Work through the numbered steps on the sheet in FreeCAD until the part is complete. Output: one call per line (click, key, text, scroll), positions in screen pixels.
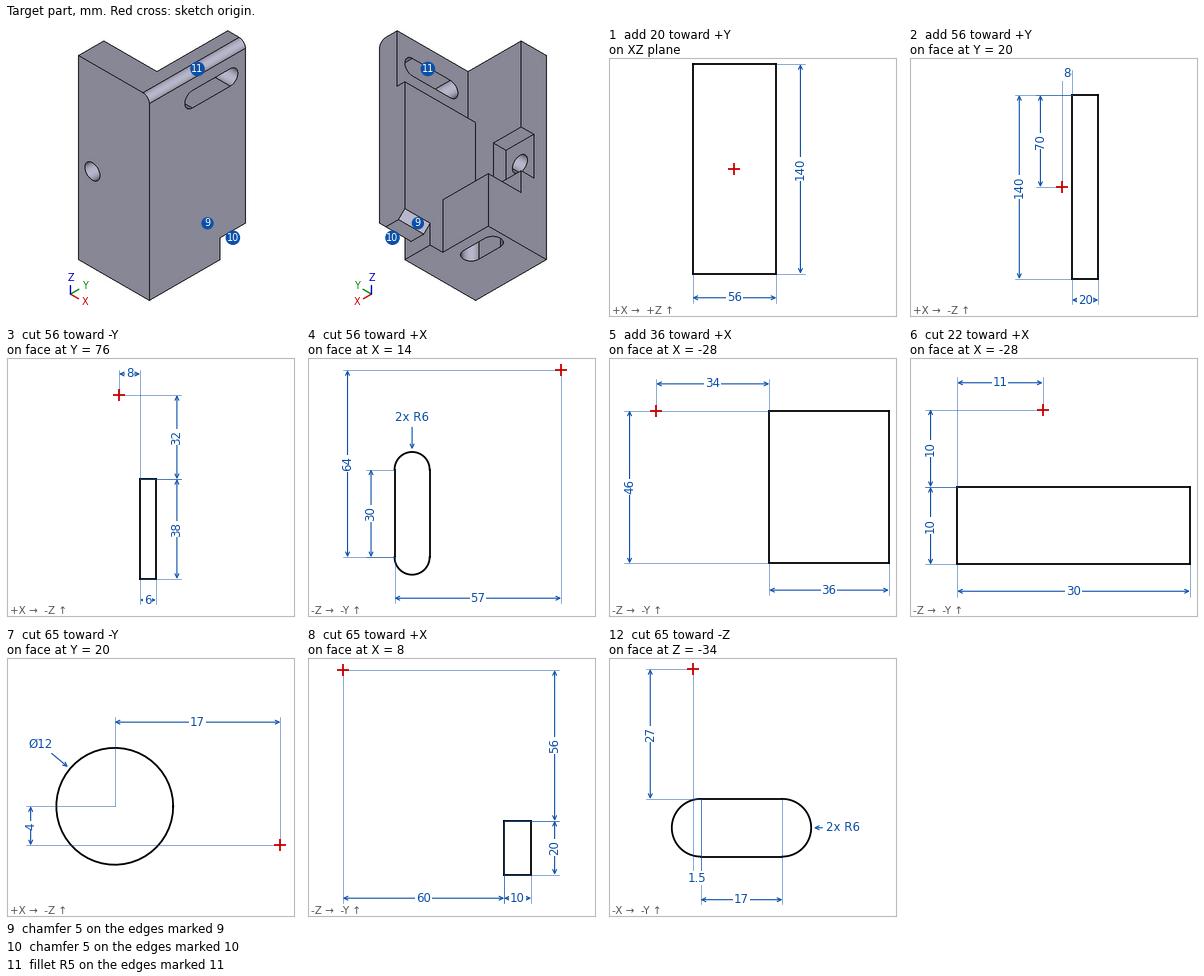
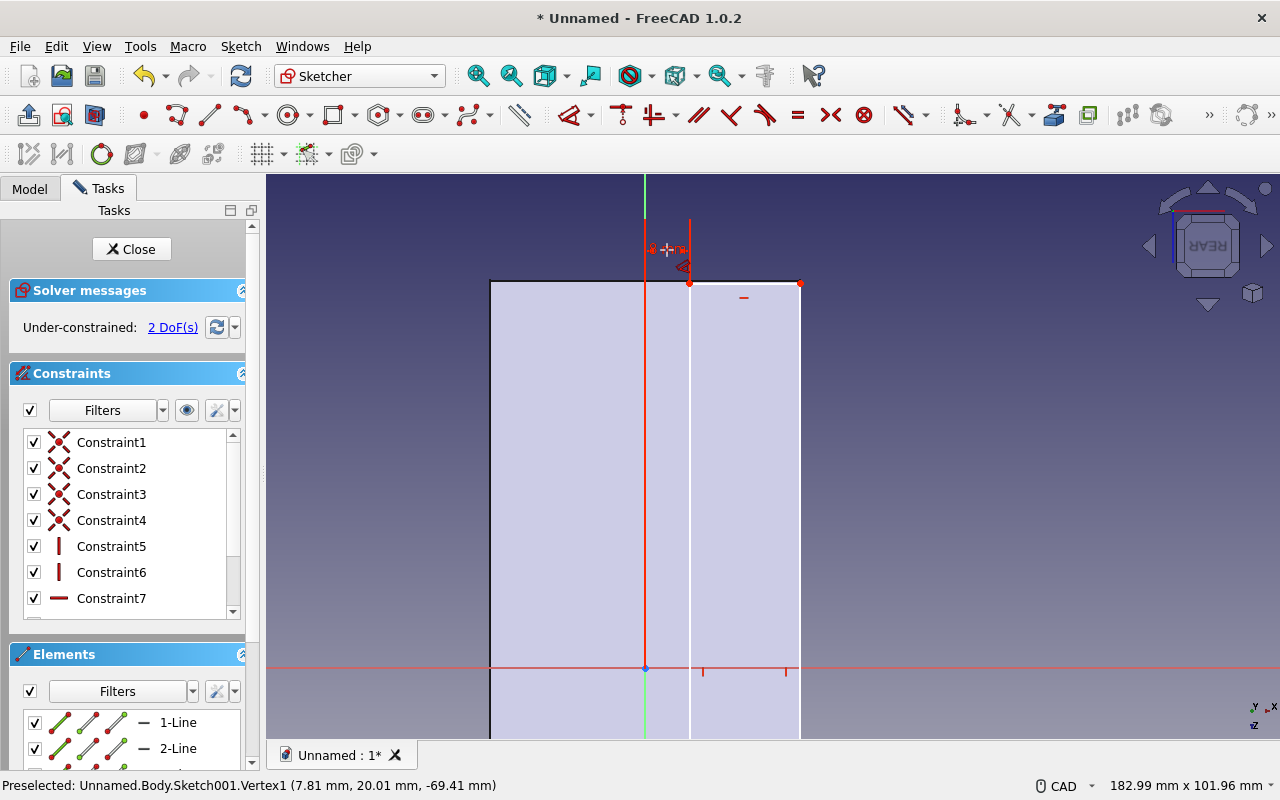
click(690, 516)
click(724, 497)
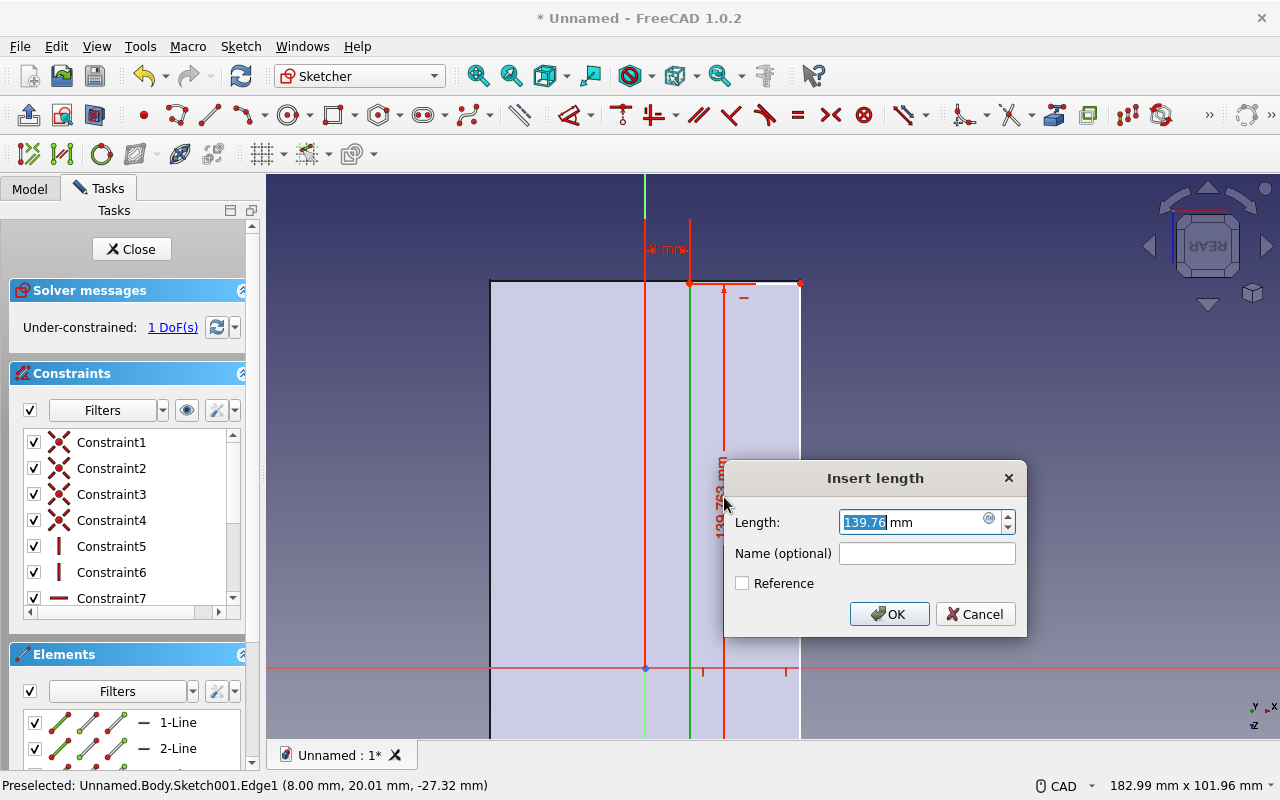
text(140)
key(Return)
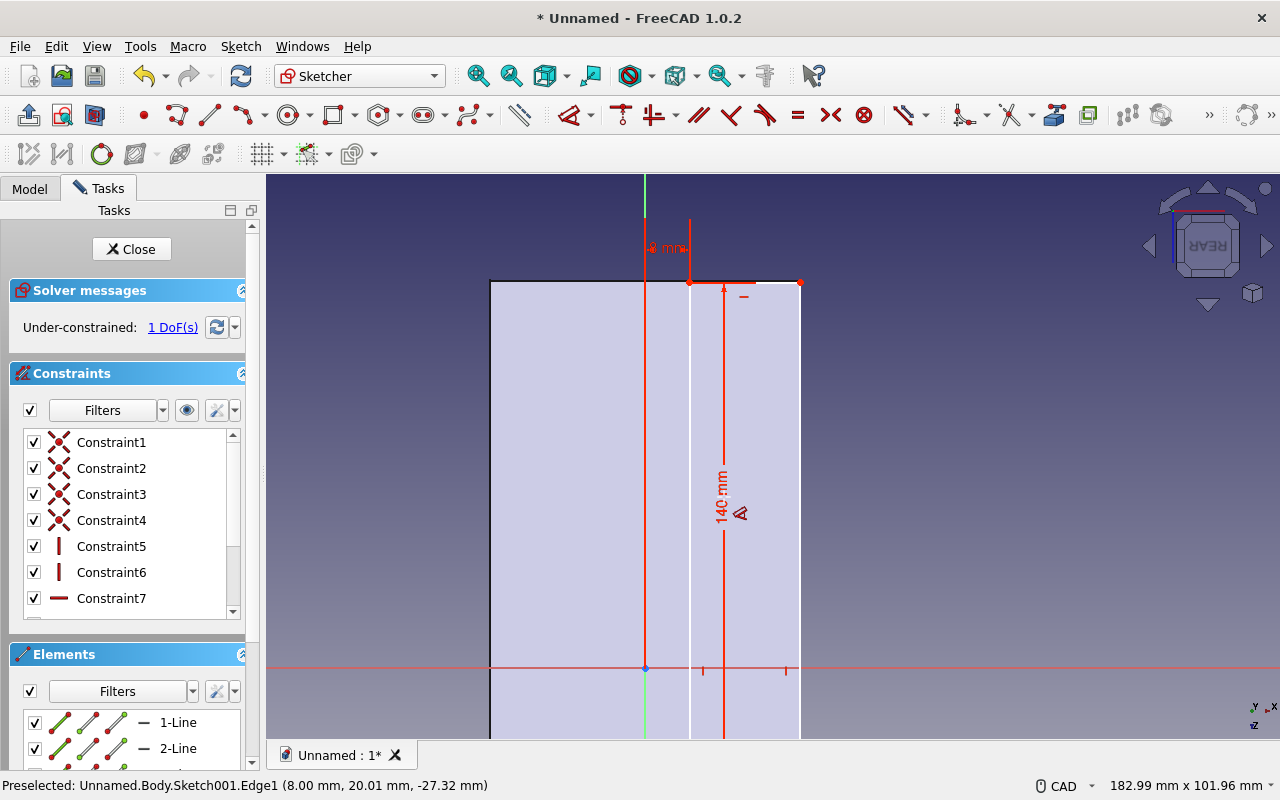
click(690, 283)
click(611, 476)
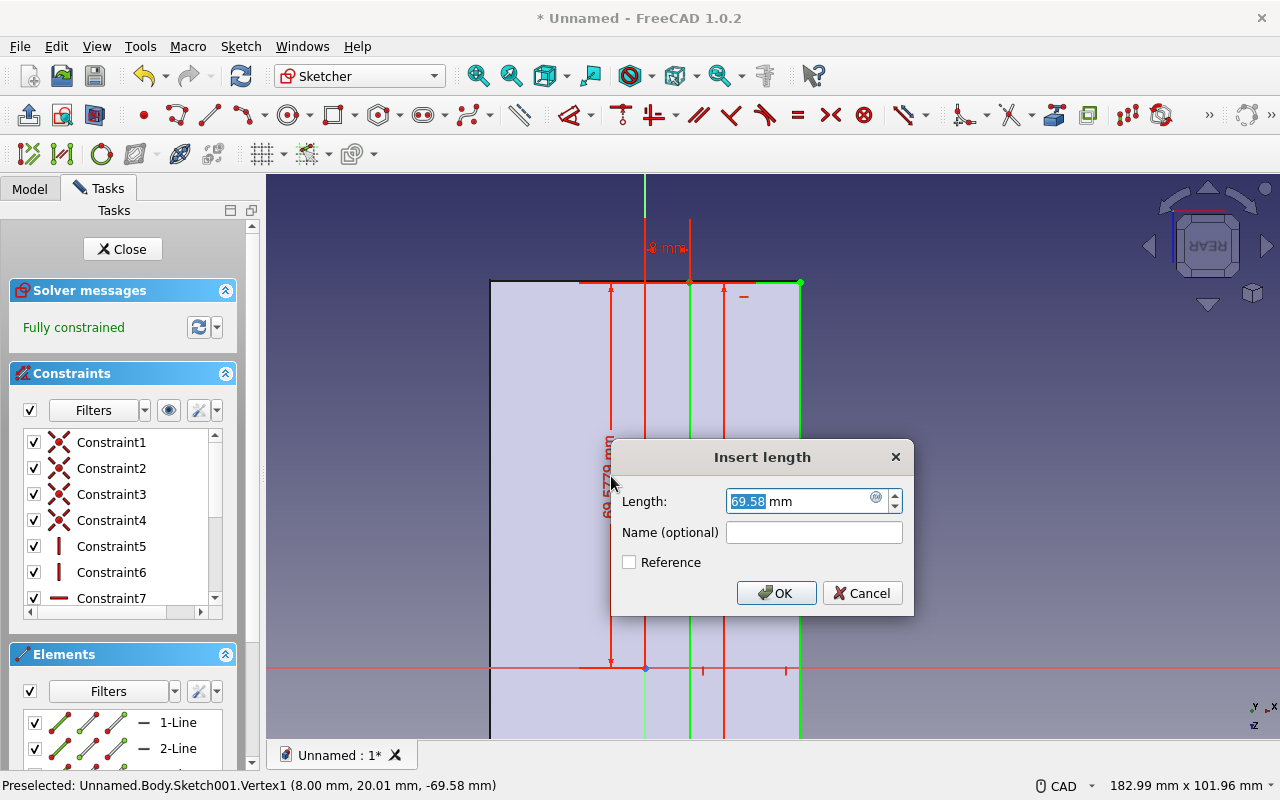
text(70)
key(Return)
key(Escape)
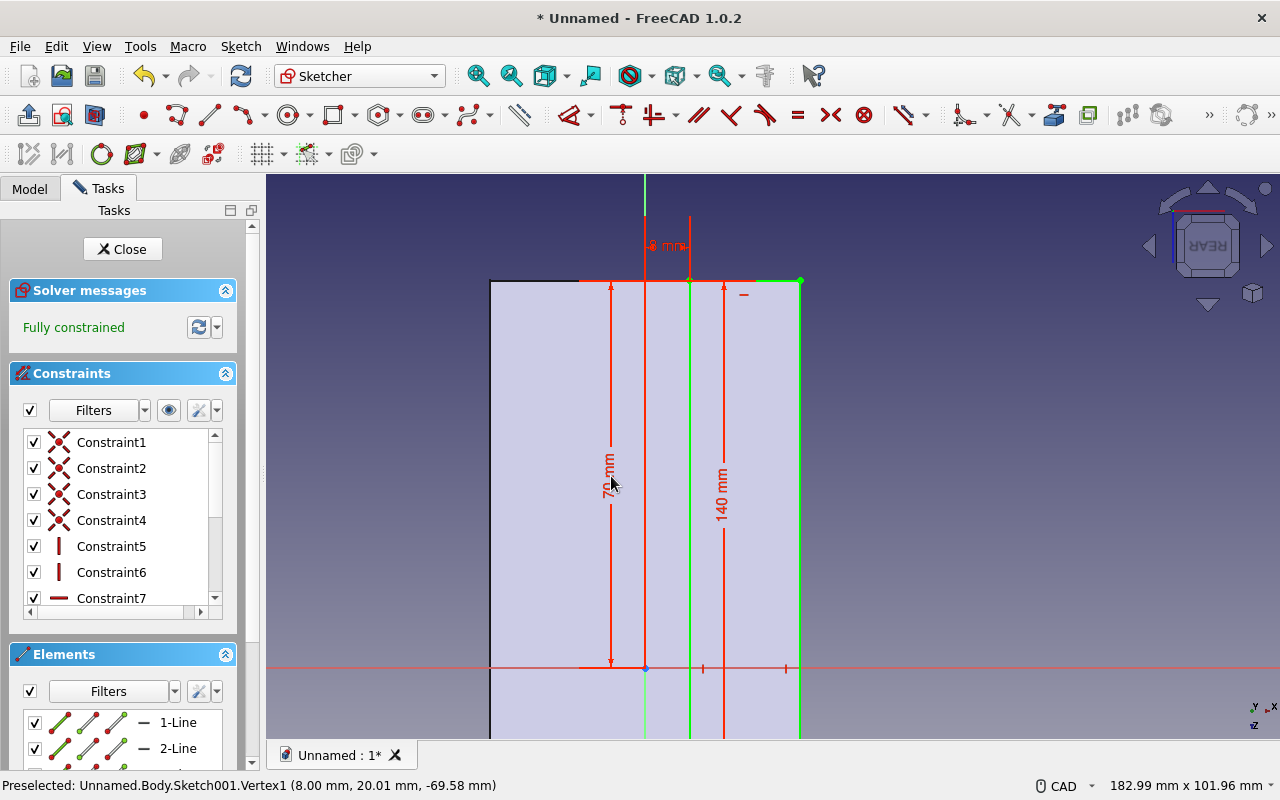
click(123, 249)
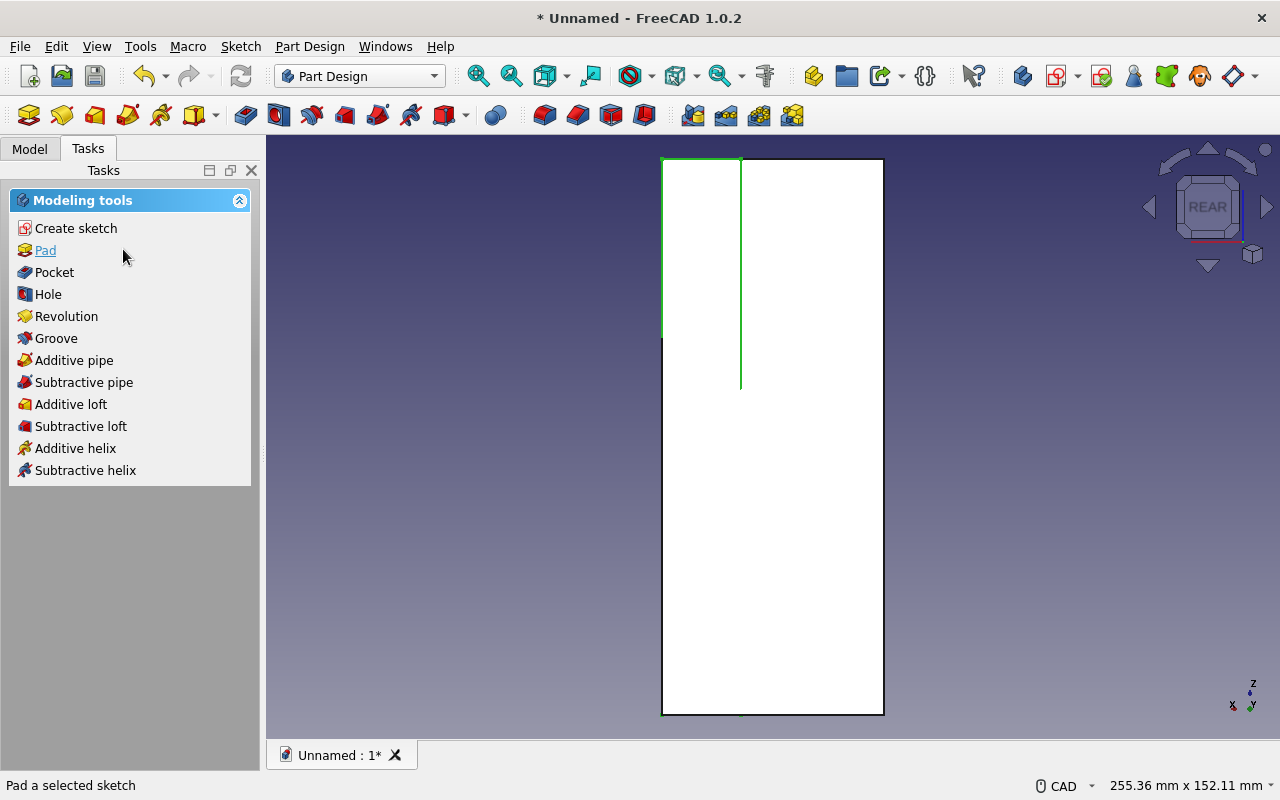
click(29, 116)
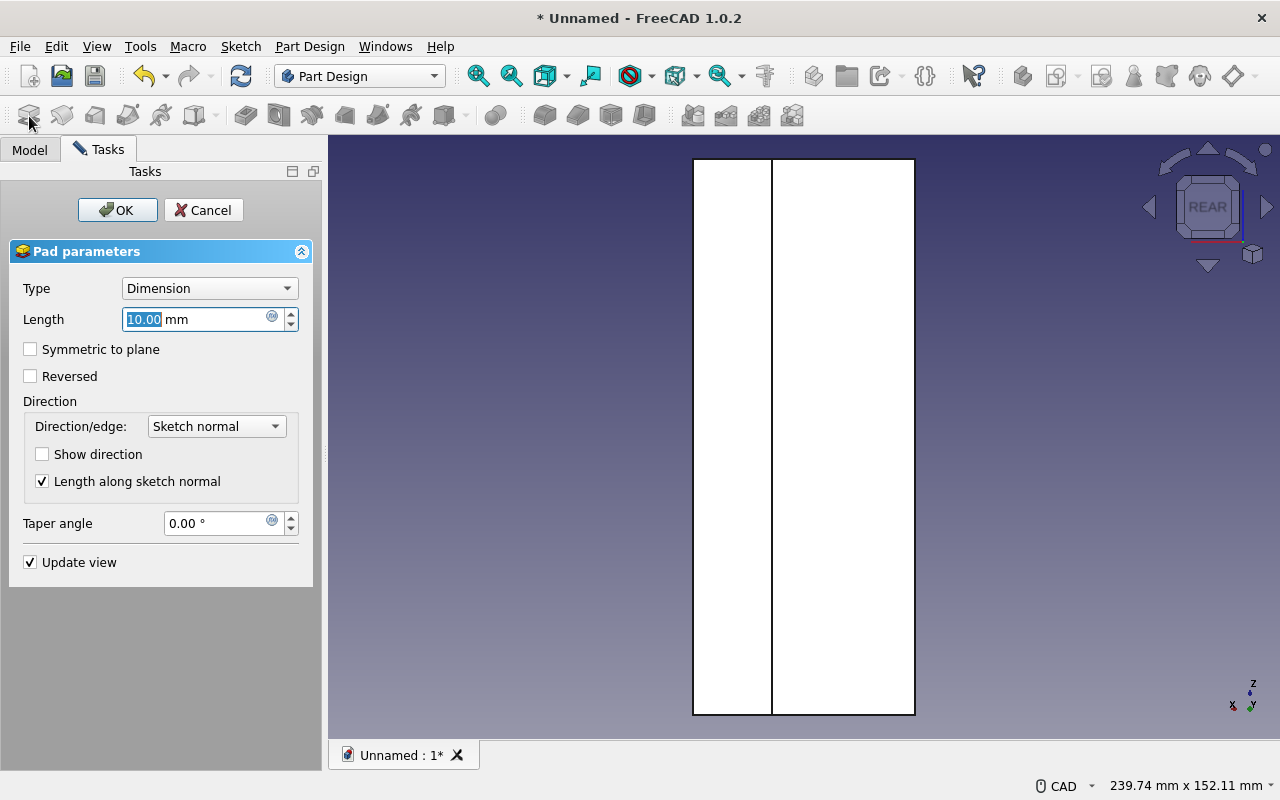
text(56)
key(Tab)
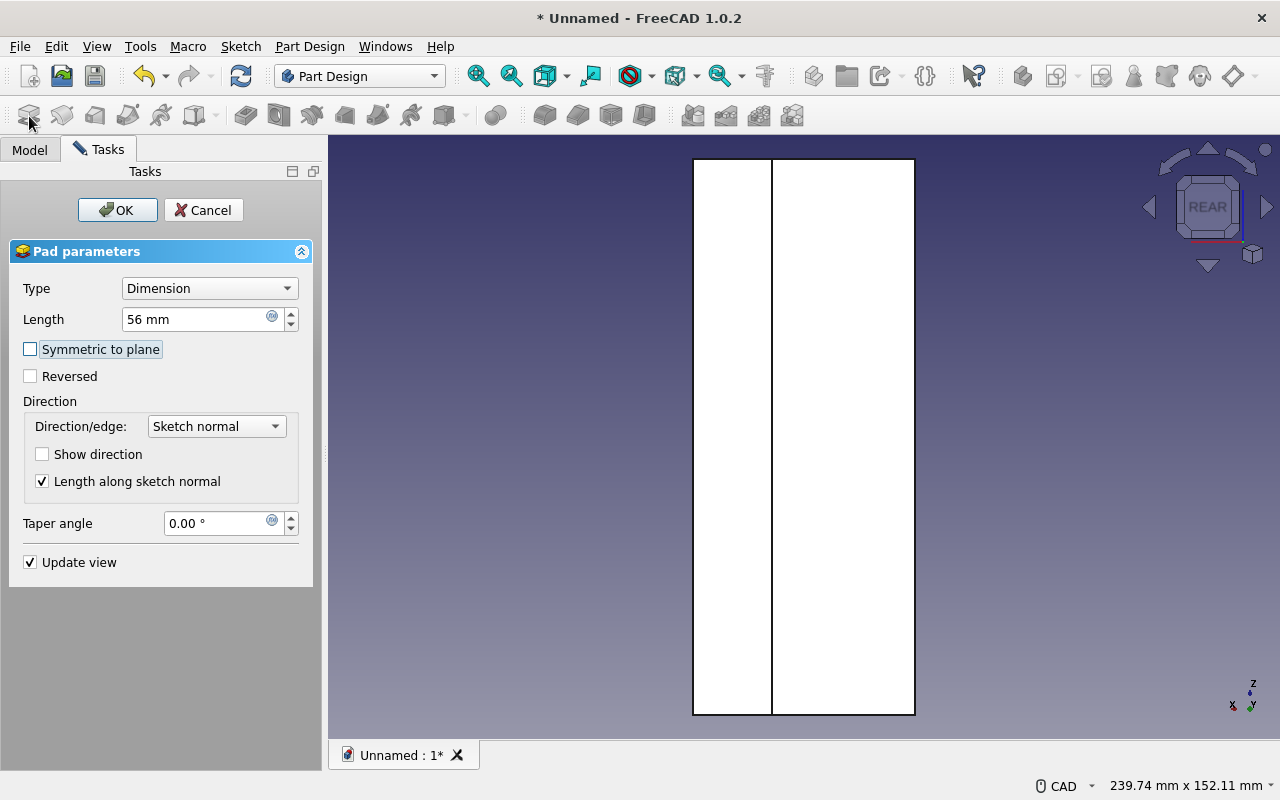
click(118, 210)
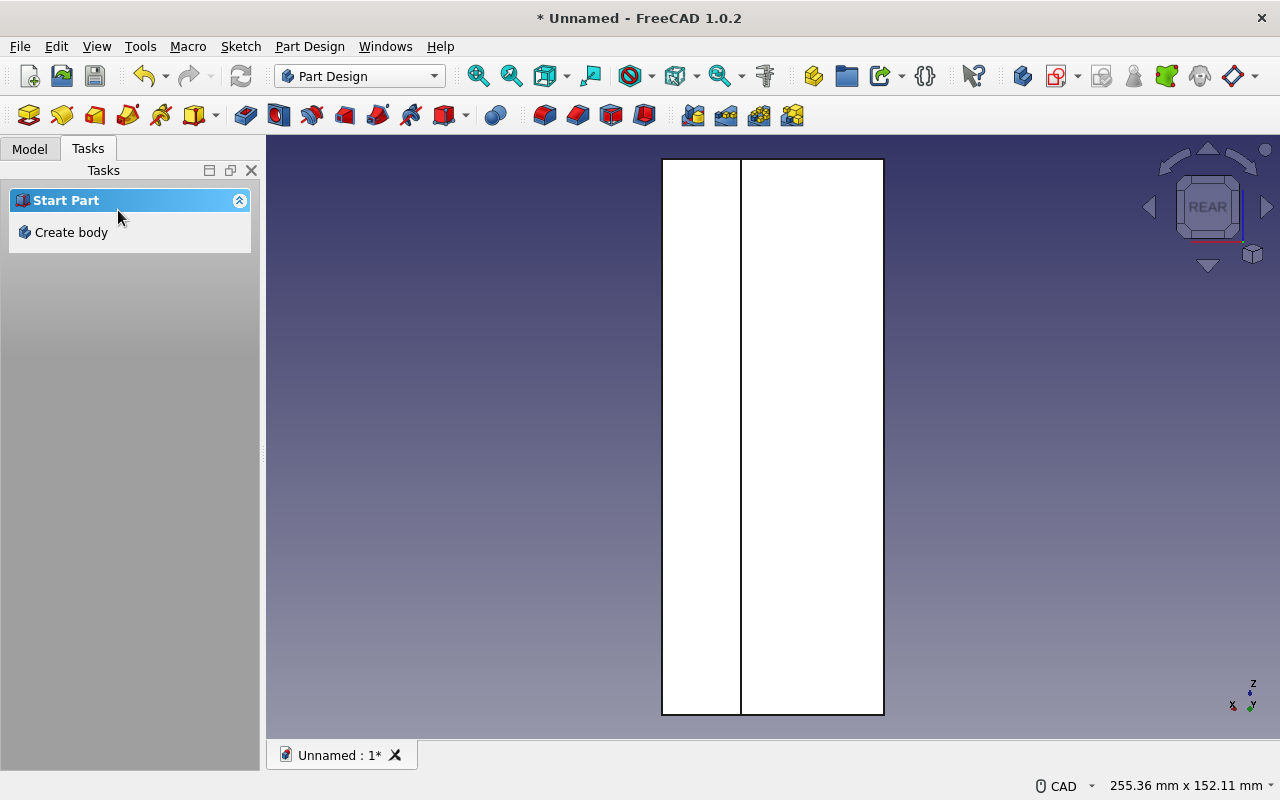
click(702, 277)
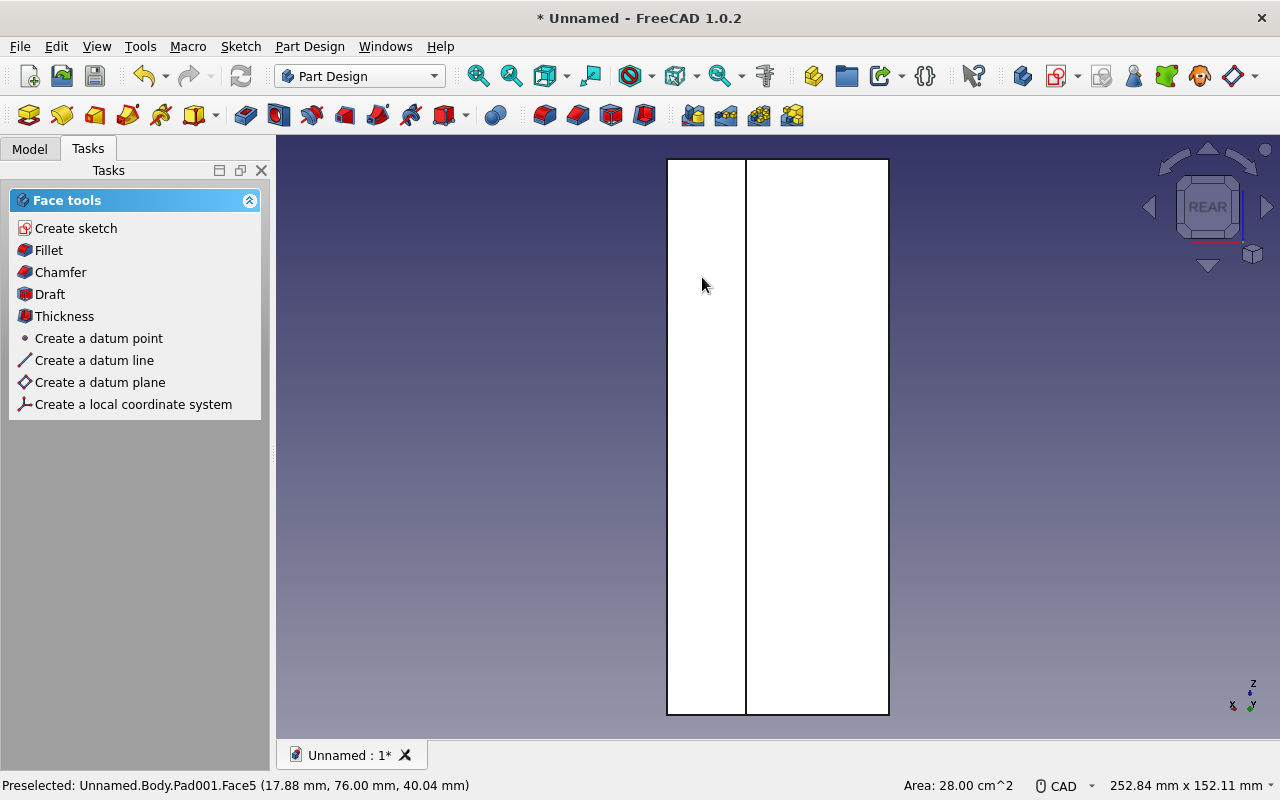
click(1056, 76)